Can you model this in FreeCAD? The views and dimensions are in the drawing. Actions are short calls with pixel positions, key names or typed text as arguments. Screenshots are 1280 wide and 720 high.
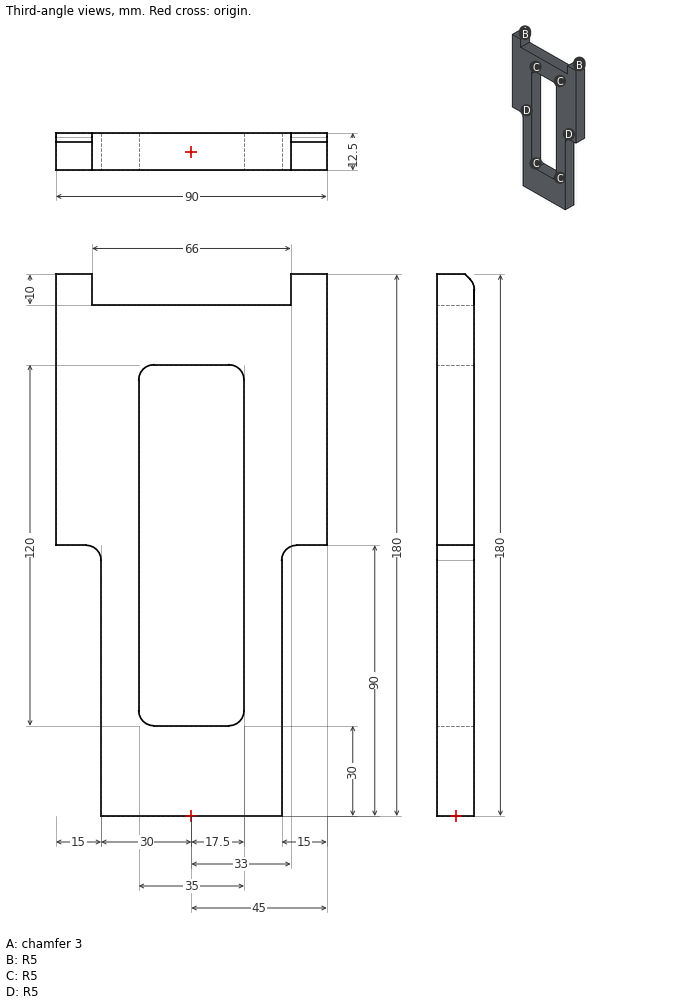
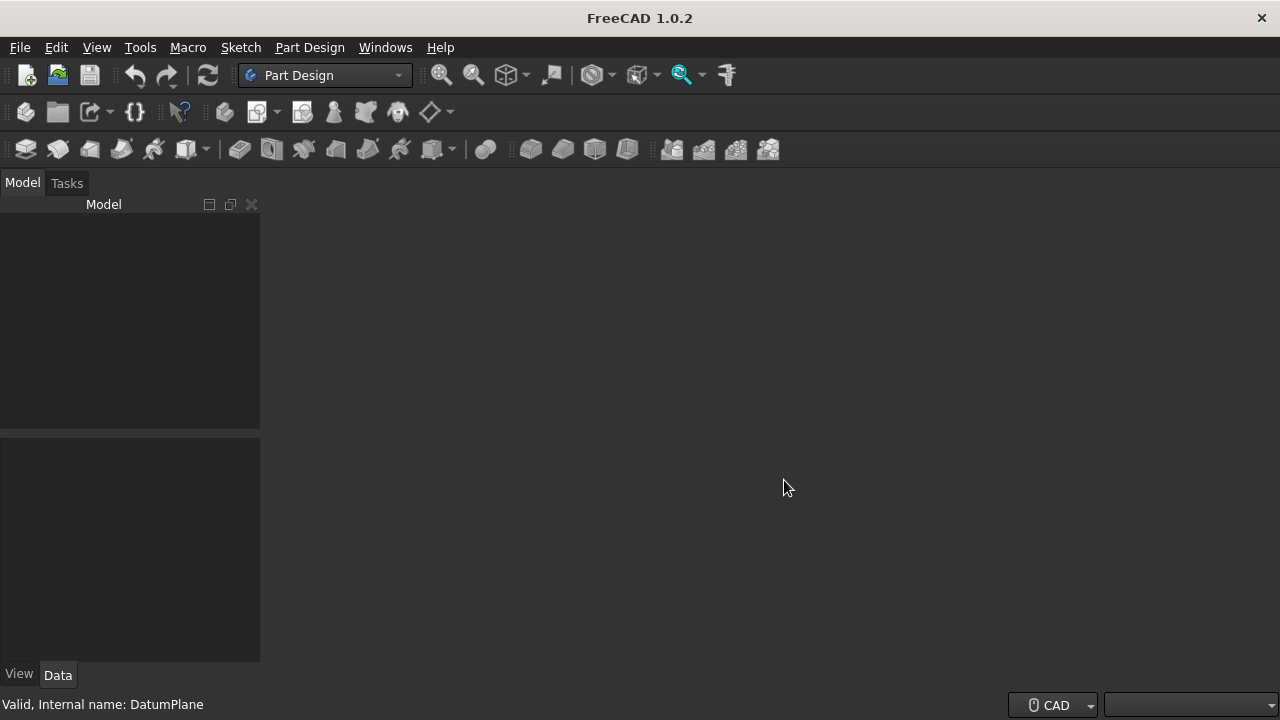
click(26, 76)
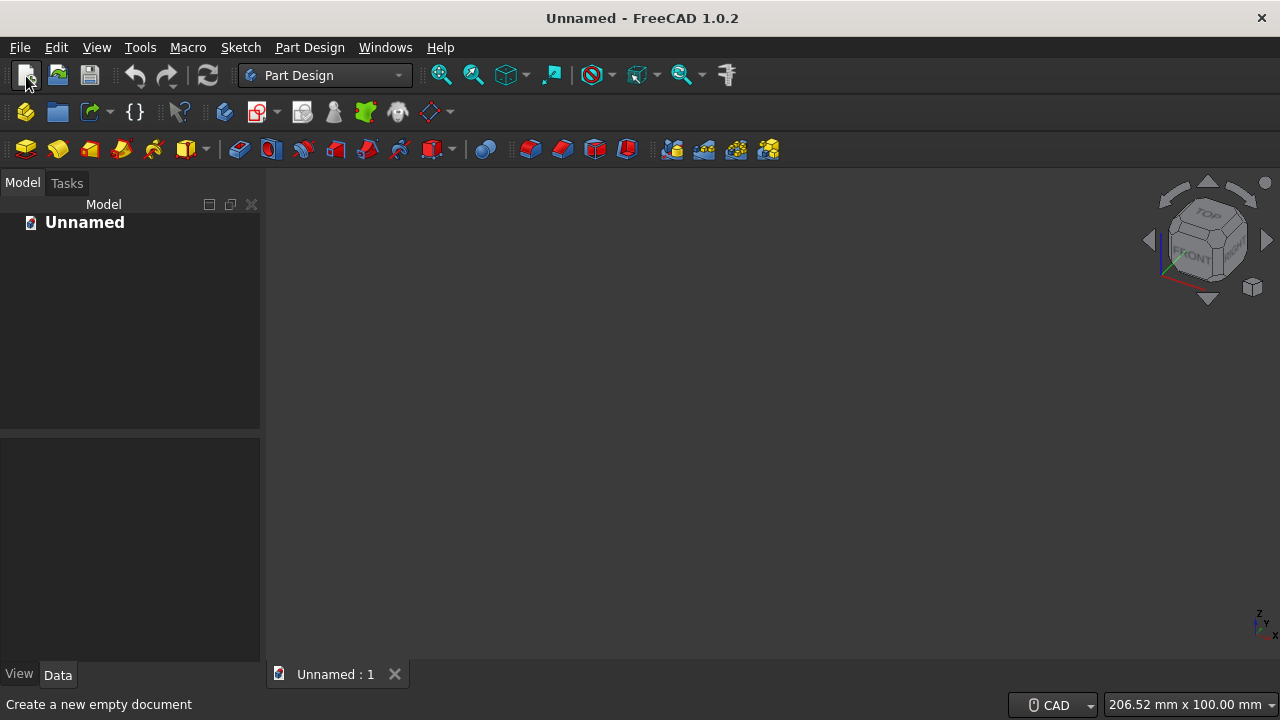
click(258, 112)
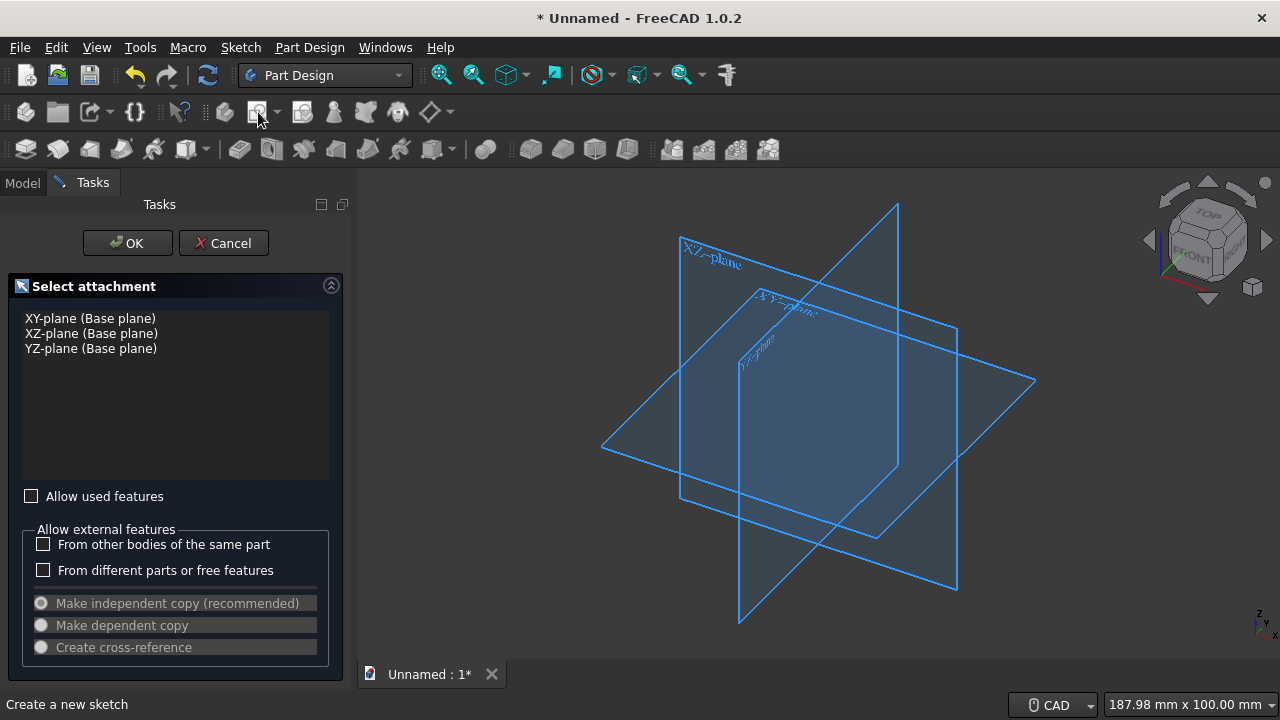
click(82, 318)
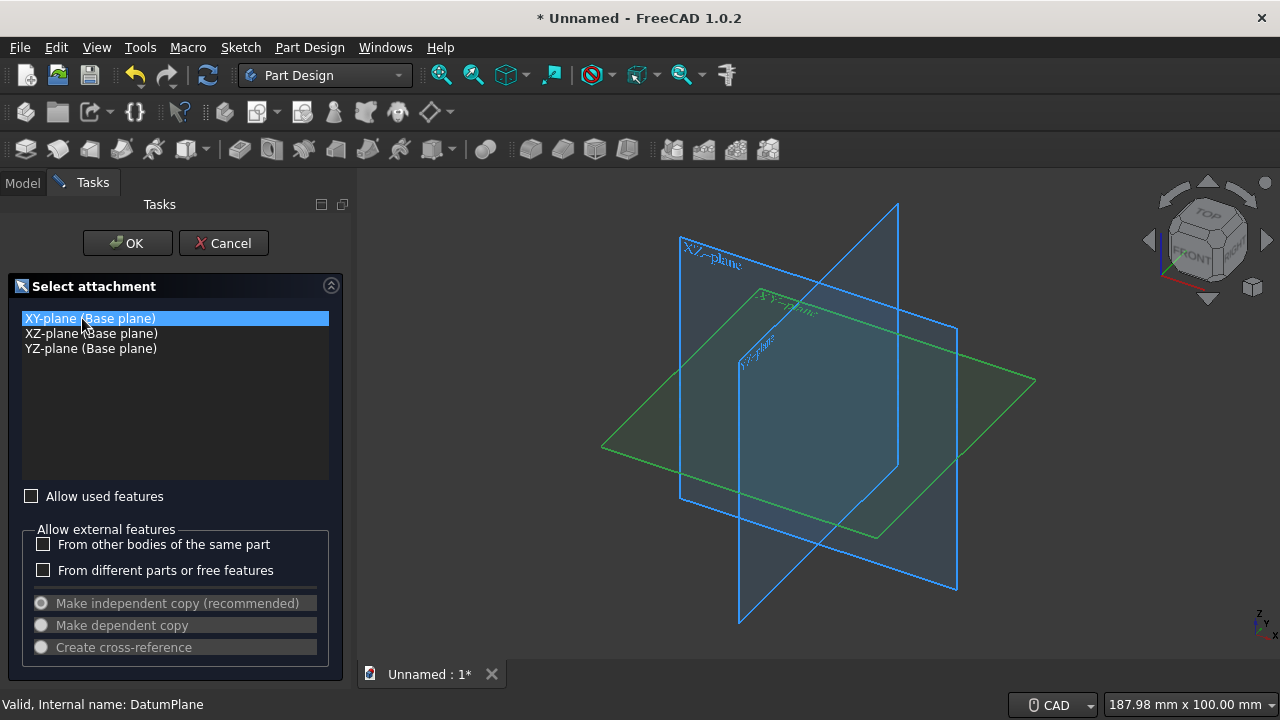
click(128, 243)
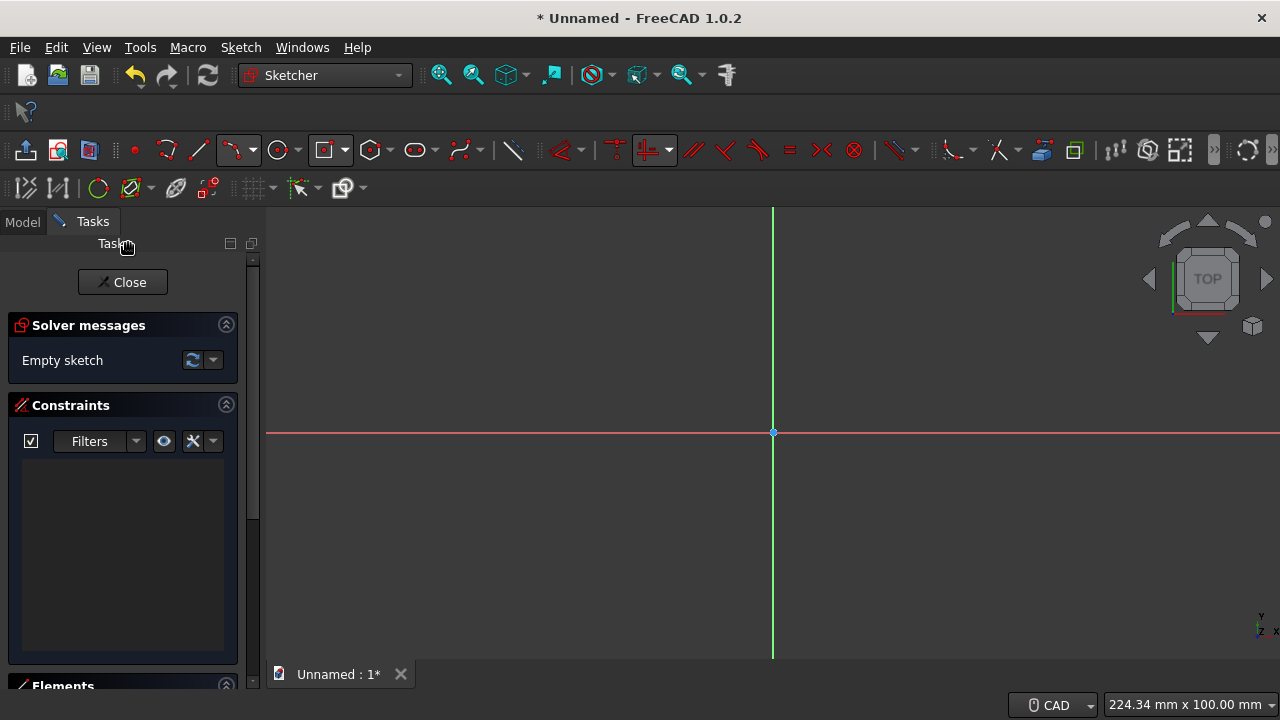
scroll(912, 433, up, 2)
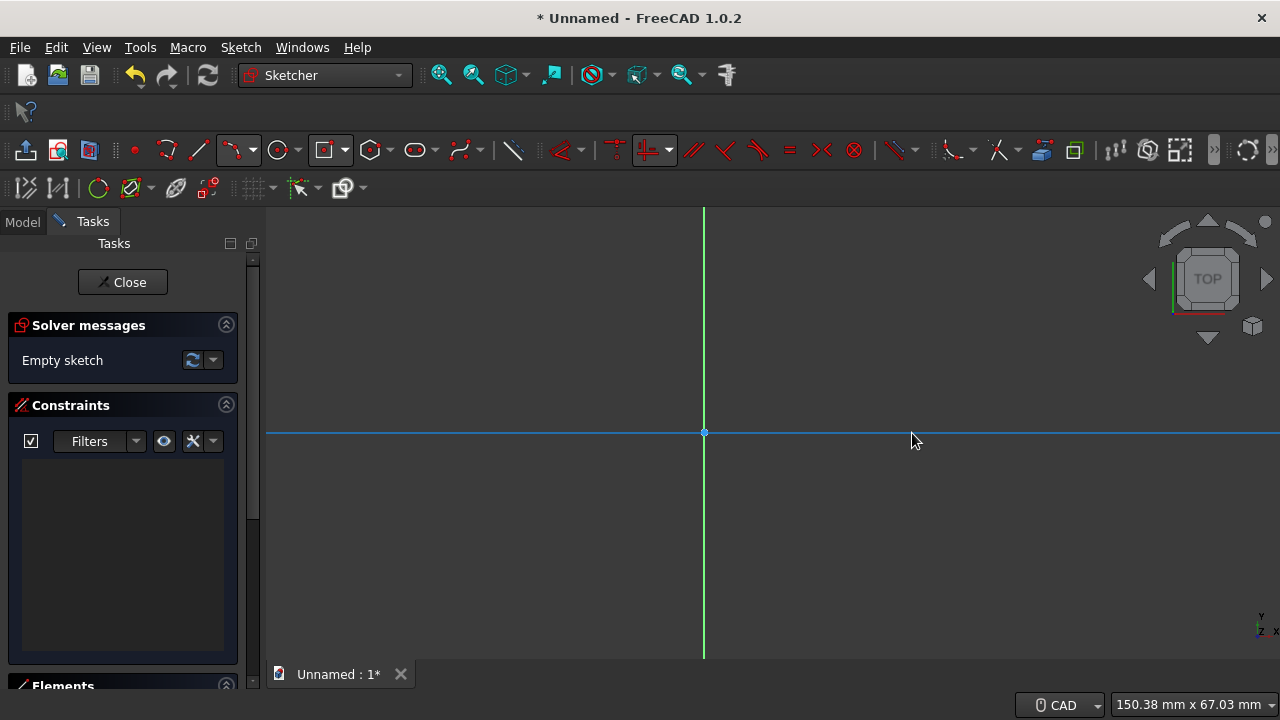
click(324, 150)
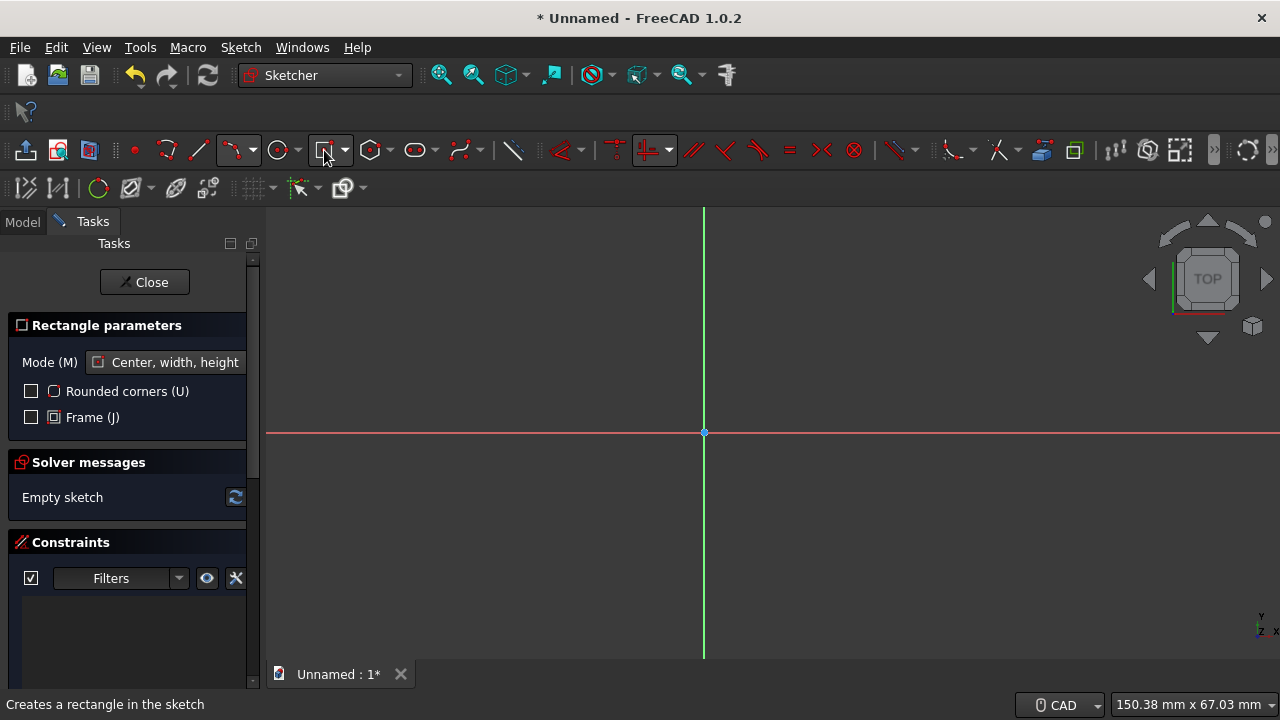
click(704, 433)
move(1008, 391)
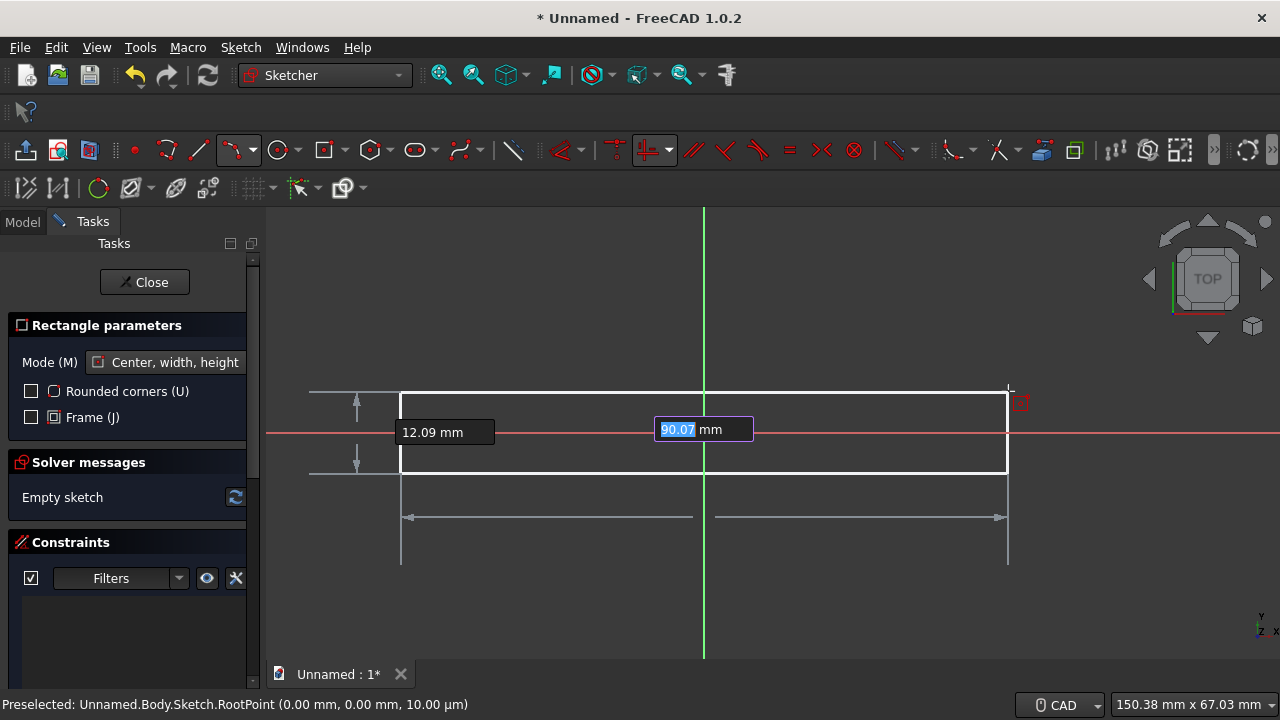
text(90)
key(Tab)
text(12.5)
key(Return)
key(Escape)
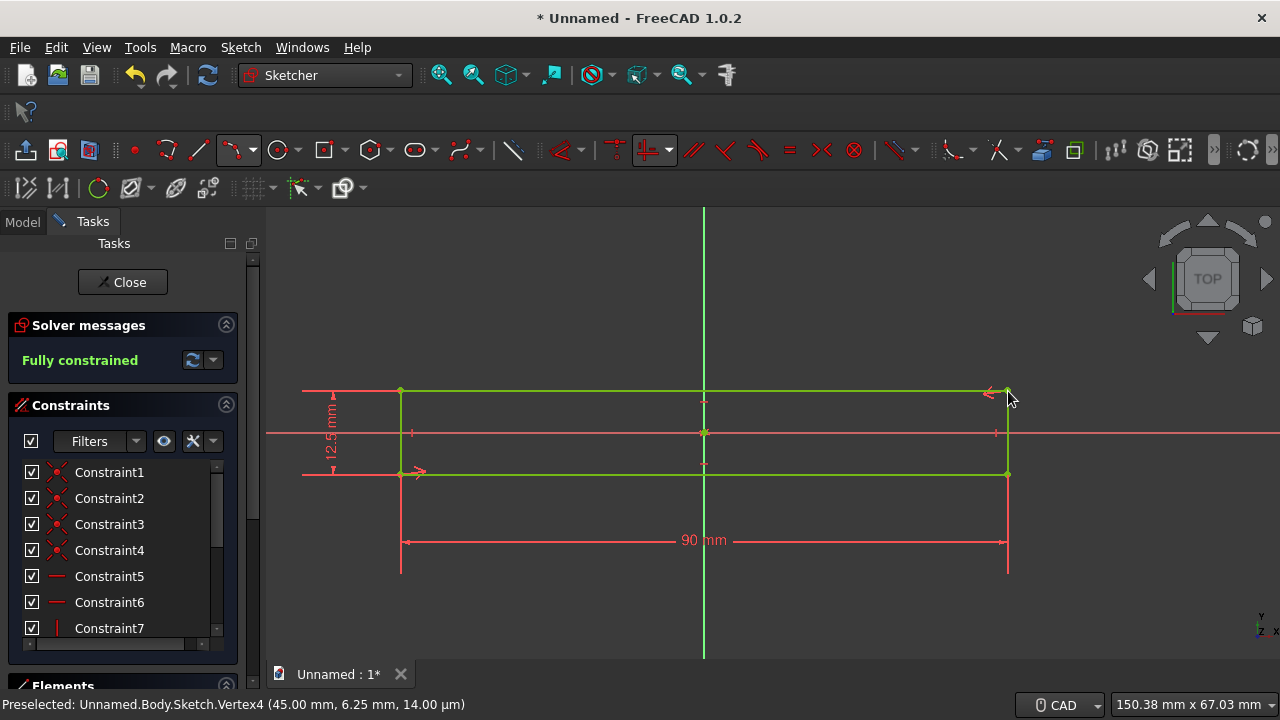
click(123, 282)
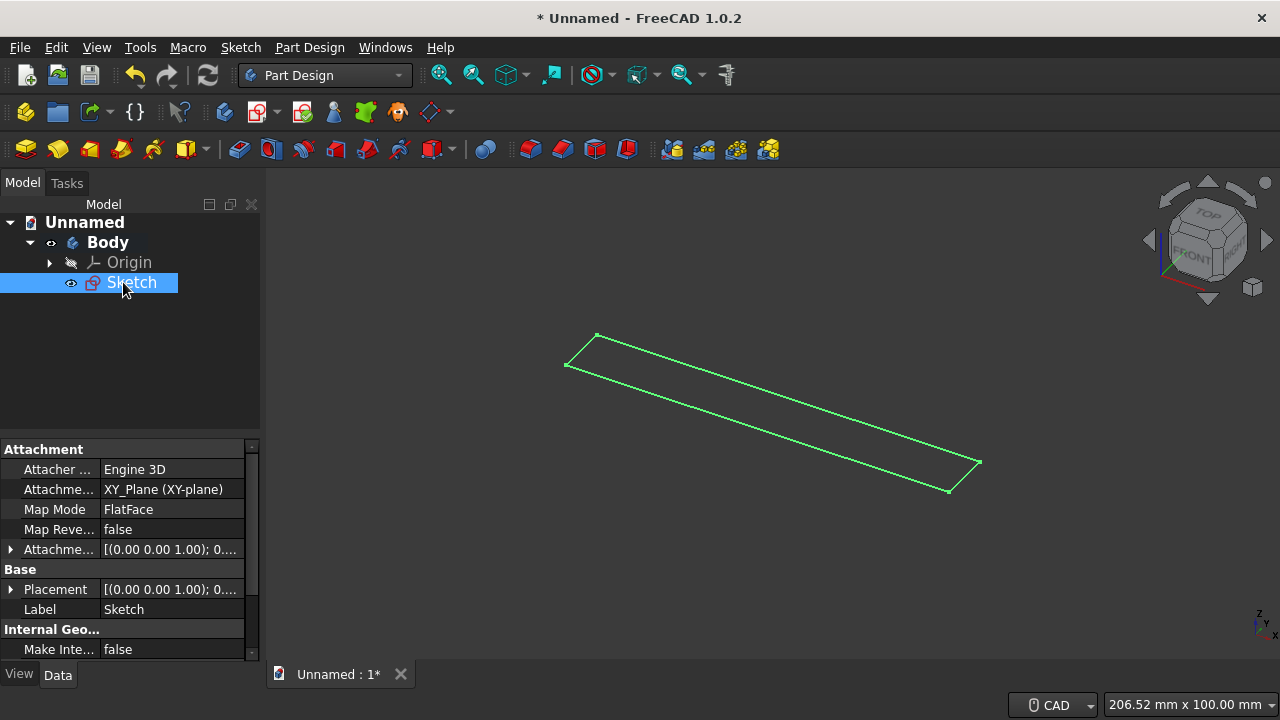
click(26, 150)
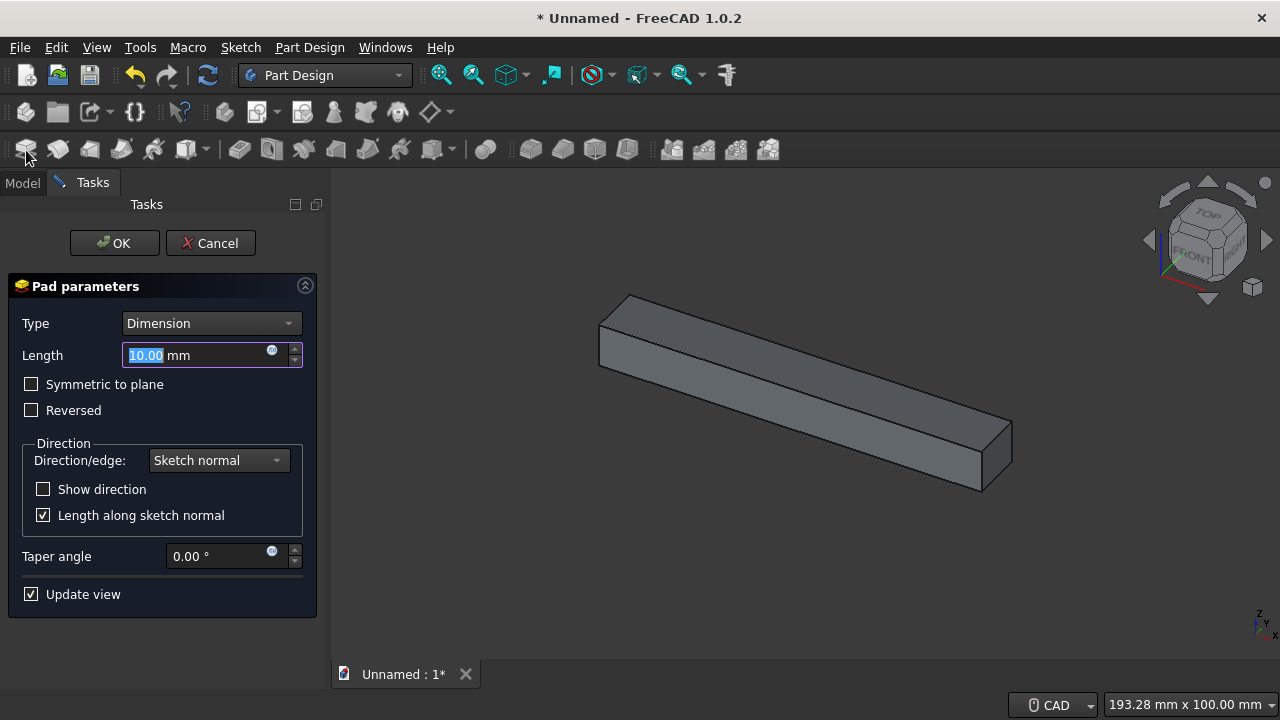
text(180)
key(Tab)